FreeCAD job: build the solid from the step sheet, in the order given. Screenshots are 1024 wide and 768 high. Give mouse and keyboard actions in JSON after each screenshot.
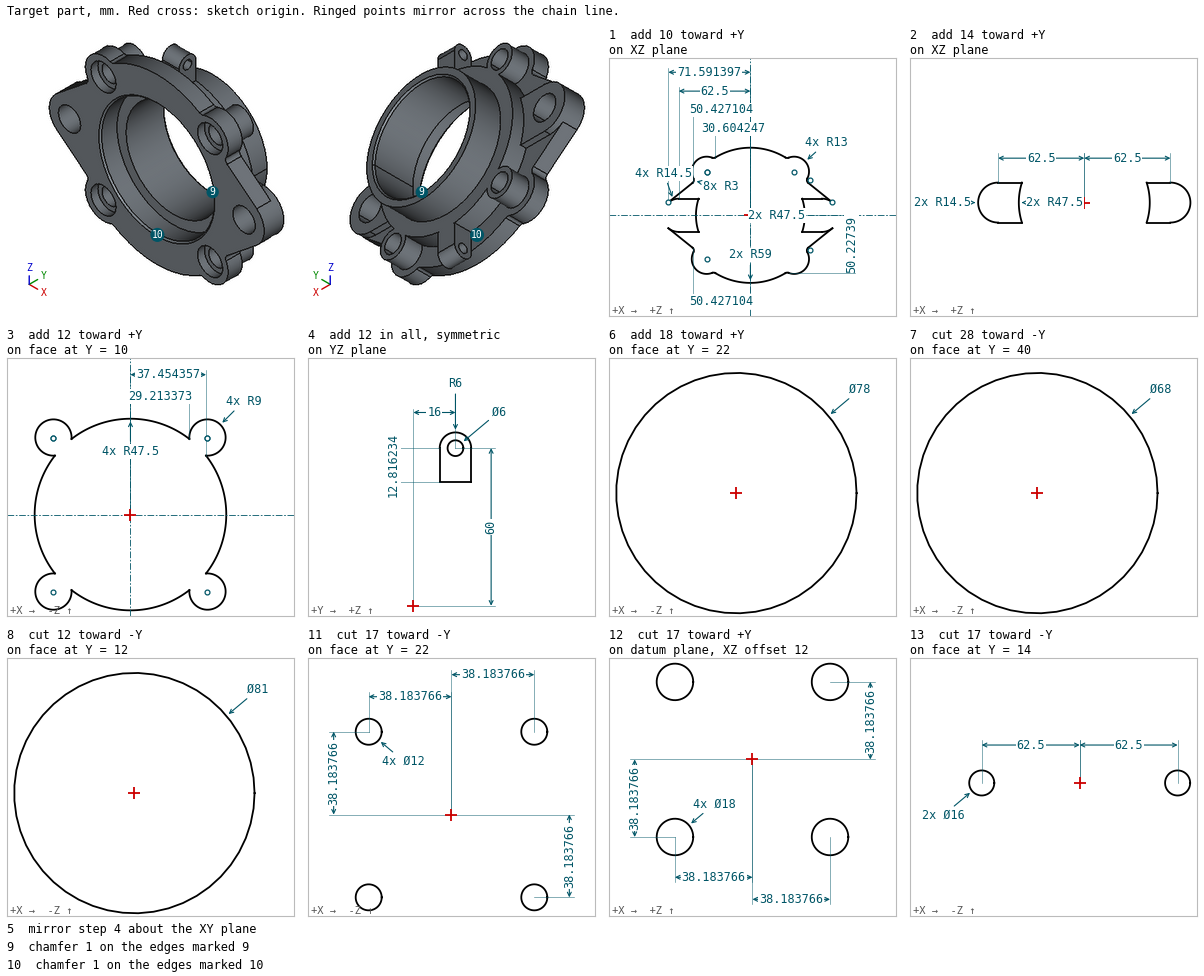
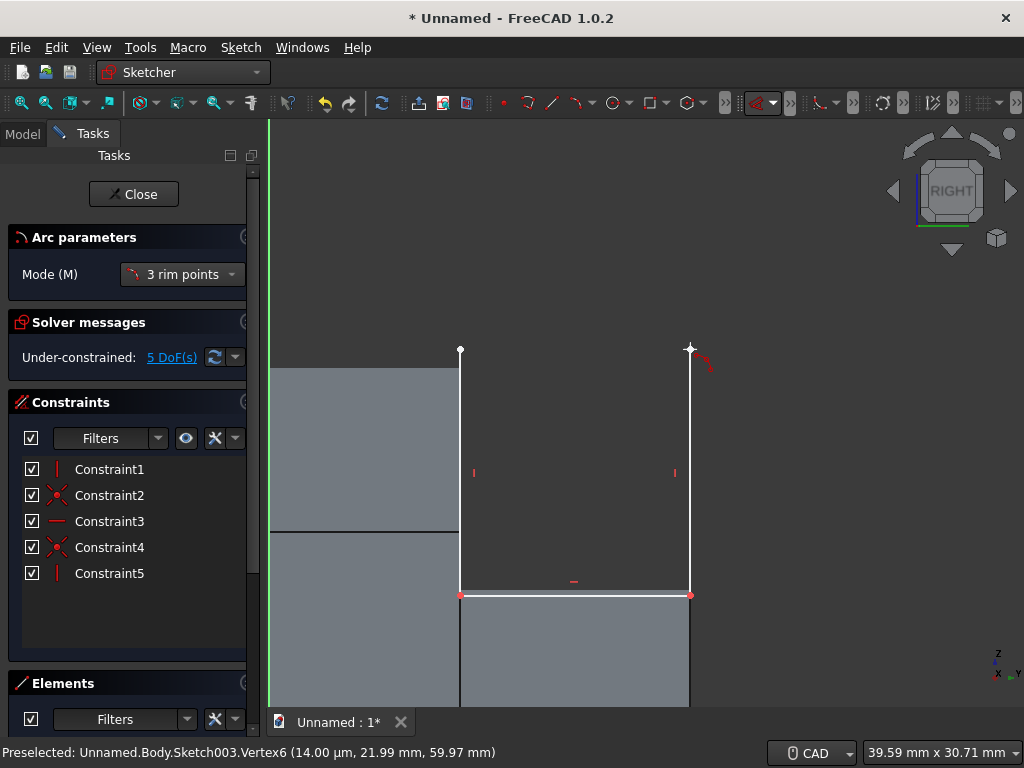
{"action": "left_click", "coordinate": [690, 350]}
{"action": "left_click", "coordinate": [460, 350]}
{"action": "left_click", "coordinate": [575, 234]}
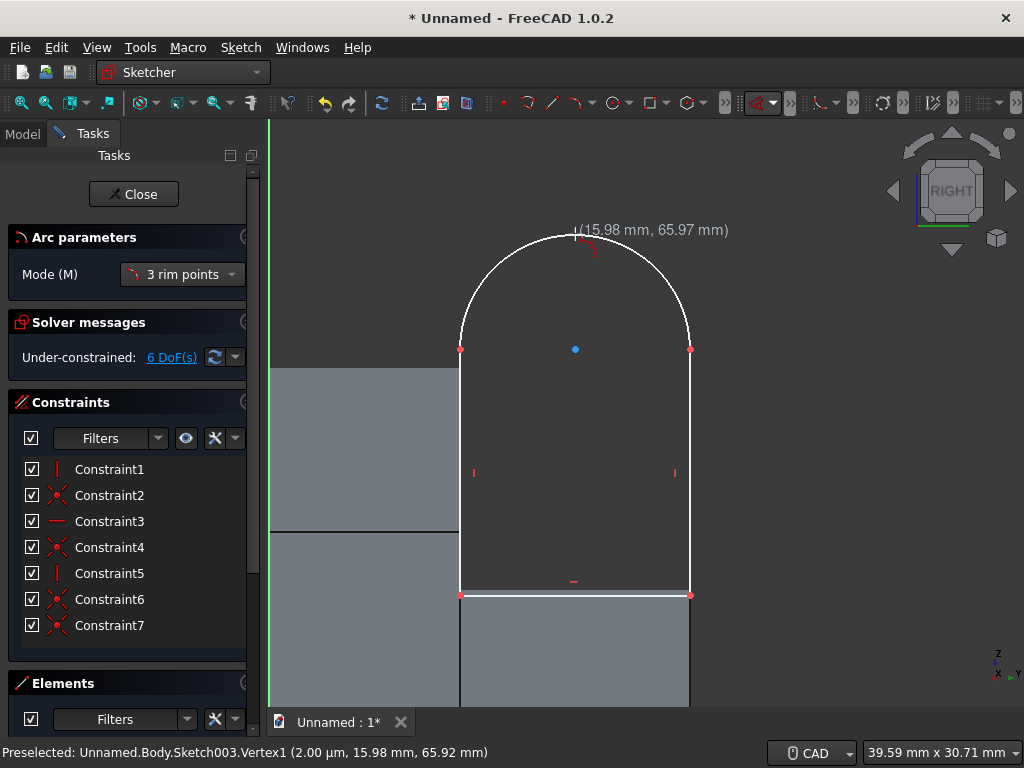
{"action": "key", "text": "g c"}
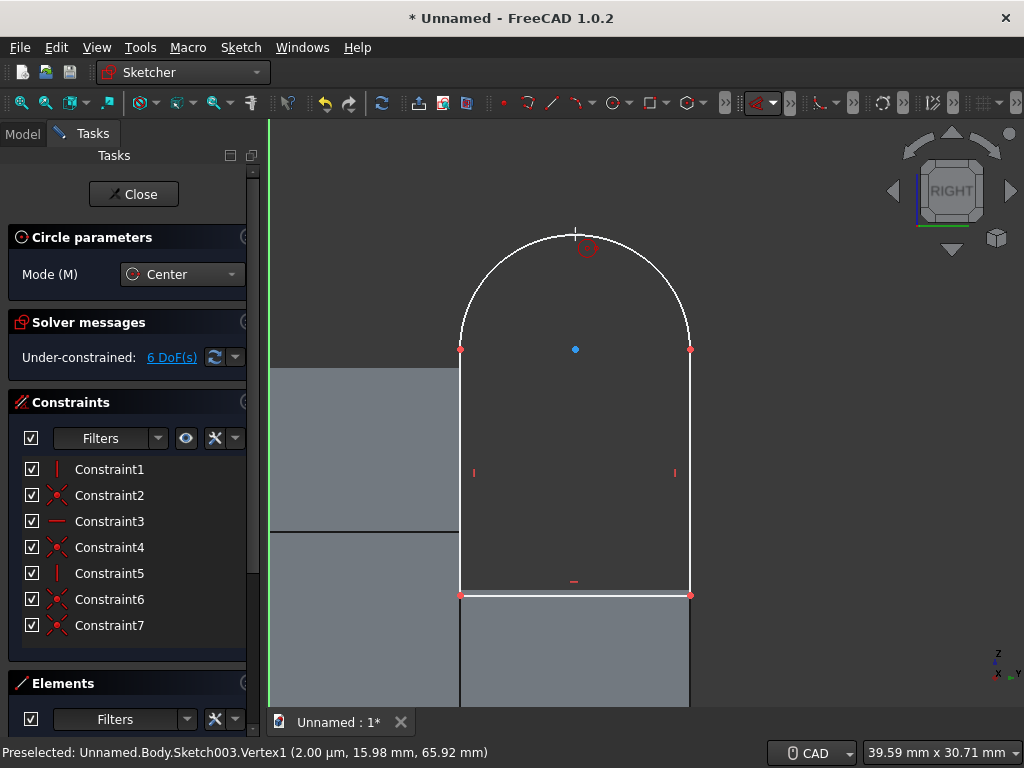
{"action": "left_click", "coordinate": [575, 349]}
{"action": "left_click", "coordinate": [616, 309]}
{"action": "key", "text": "Escape"}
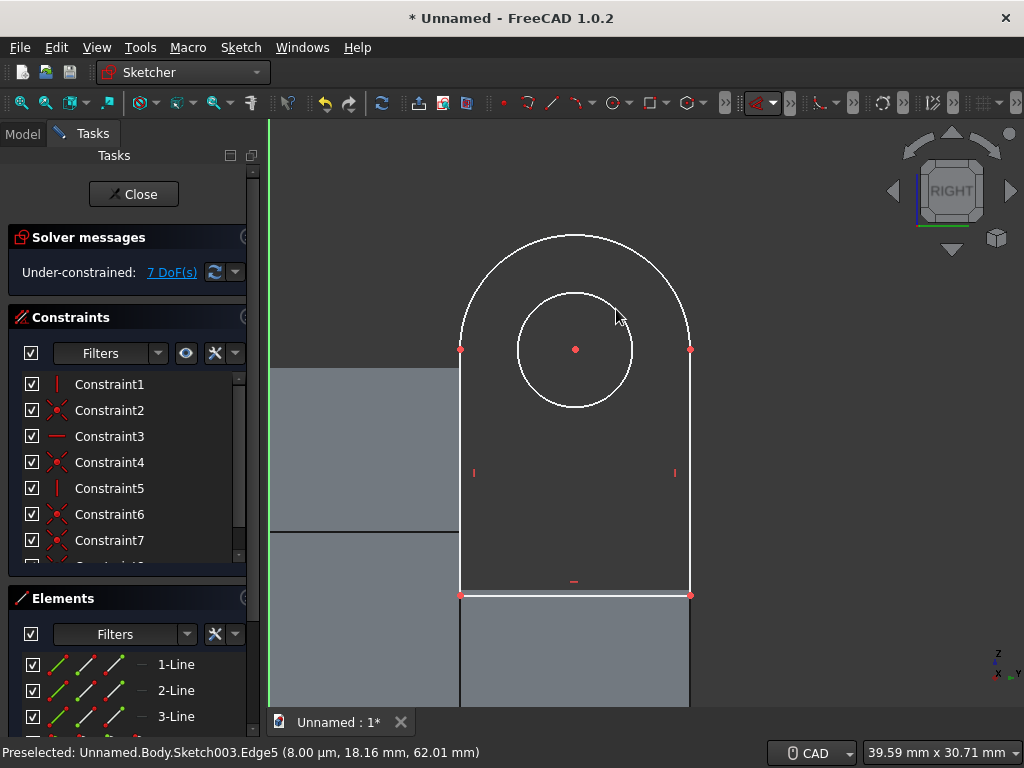
{"action": "left_click", "coordinate": [460, 424]}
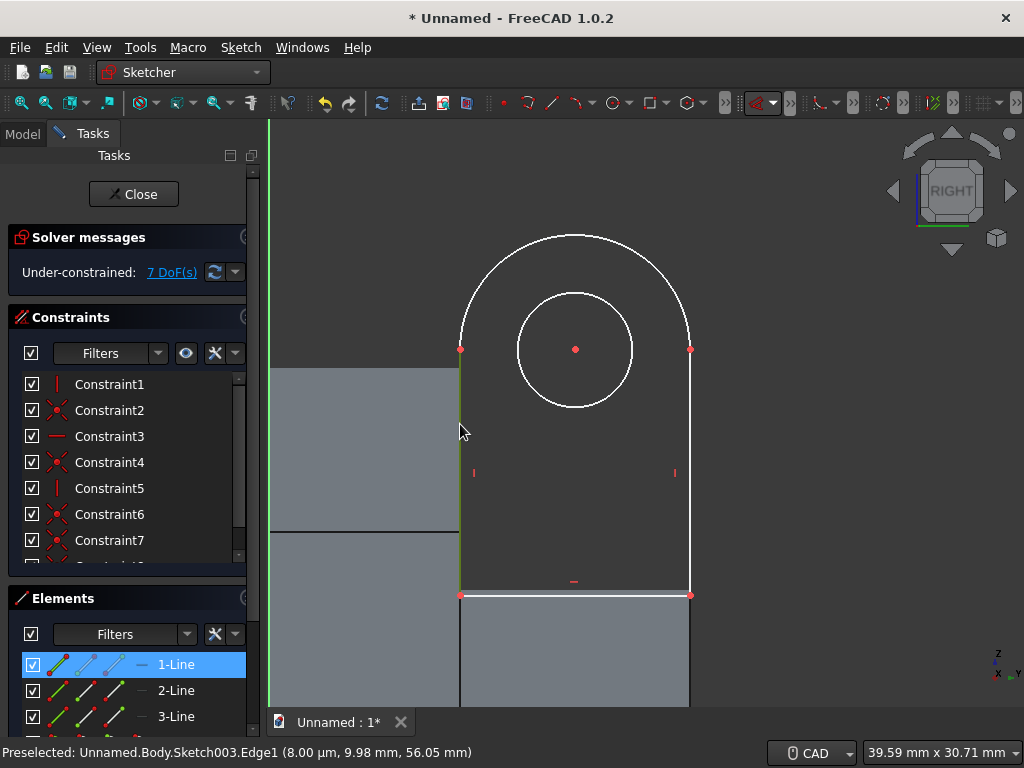
{"action": "left_click", "coordinate": [643, 257]}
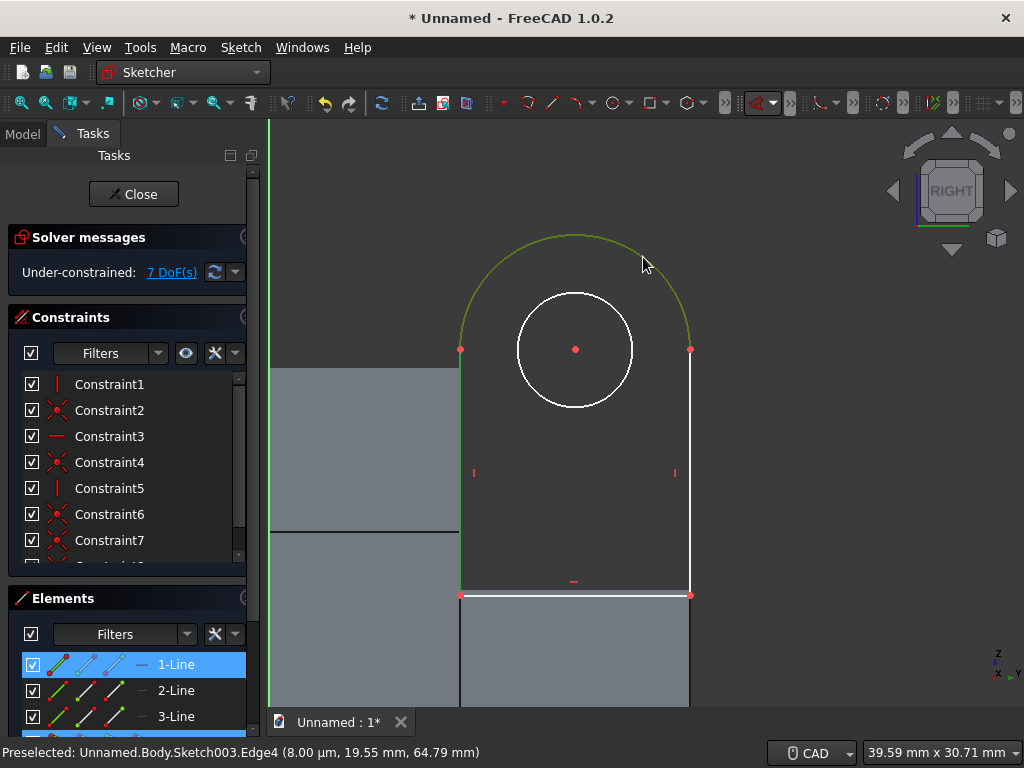
{"action": "key", "text": "t"}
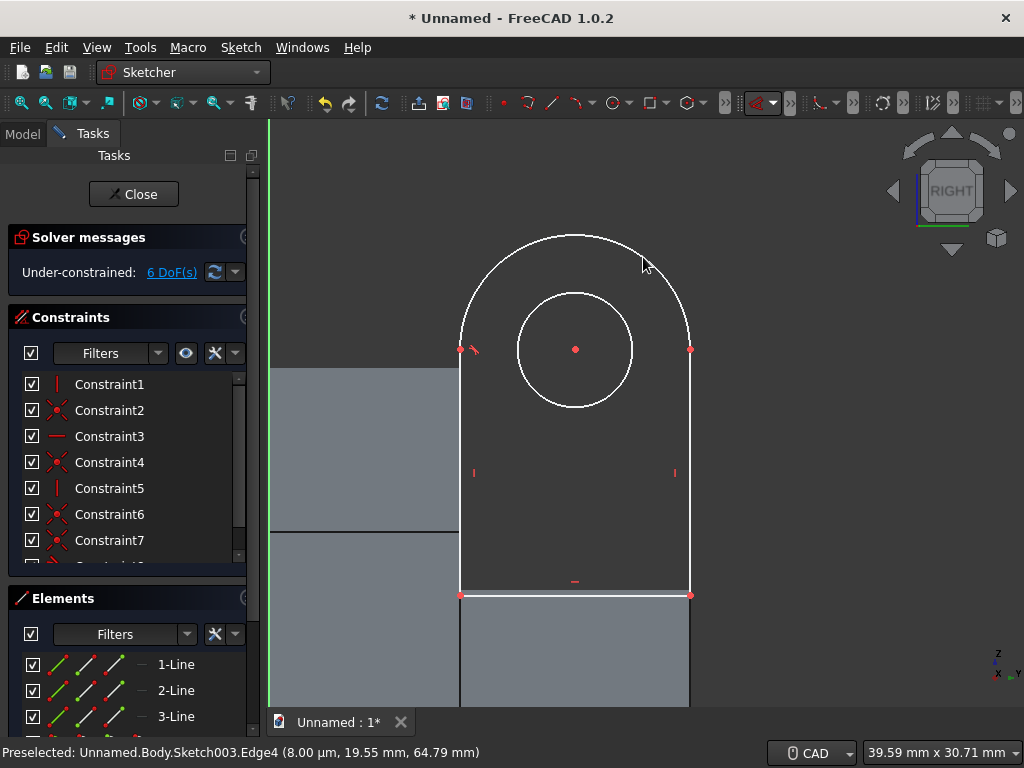
{"action": "left_click", "coordinate": [690, 522]}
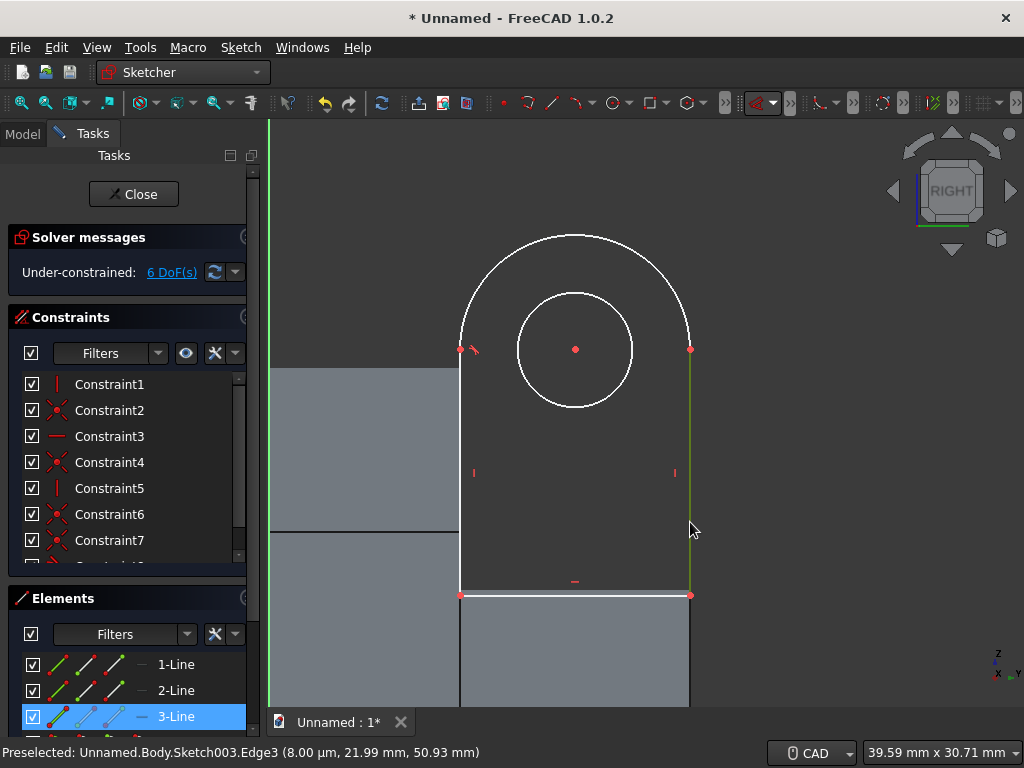
{"action": "left_click", "coordinate": [643, 257]}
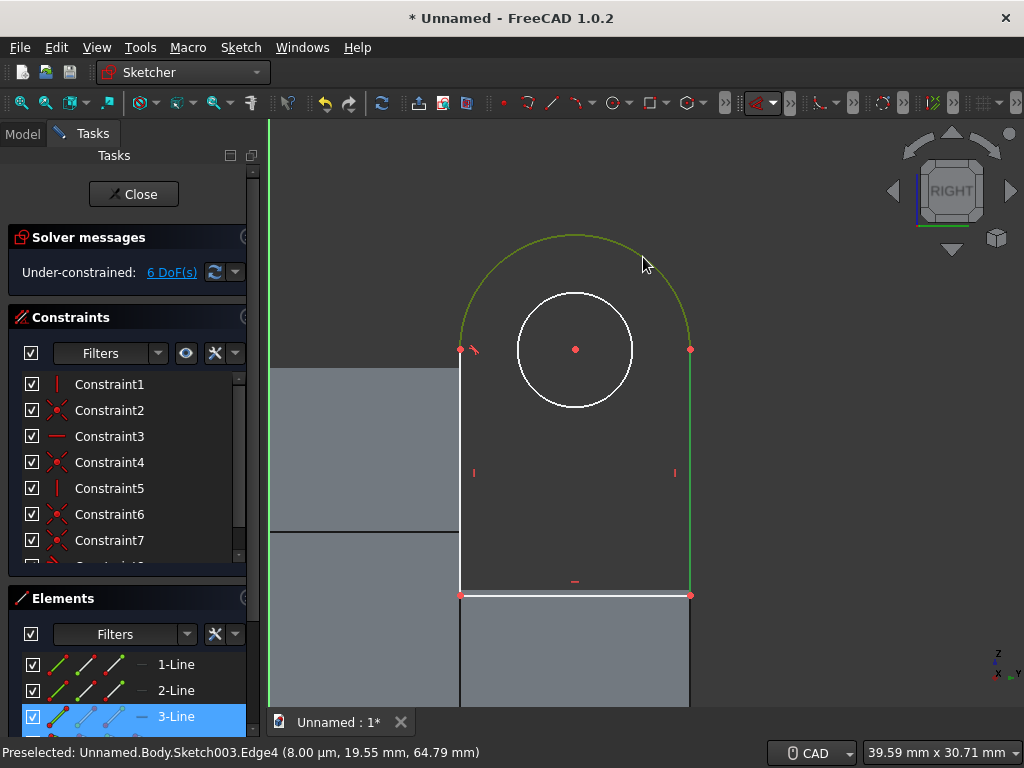
{"action": "key", "text": "t"}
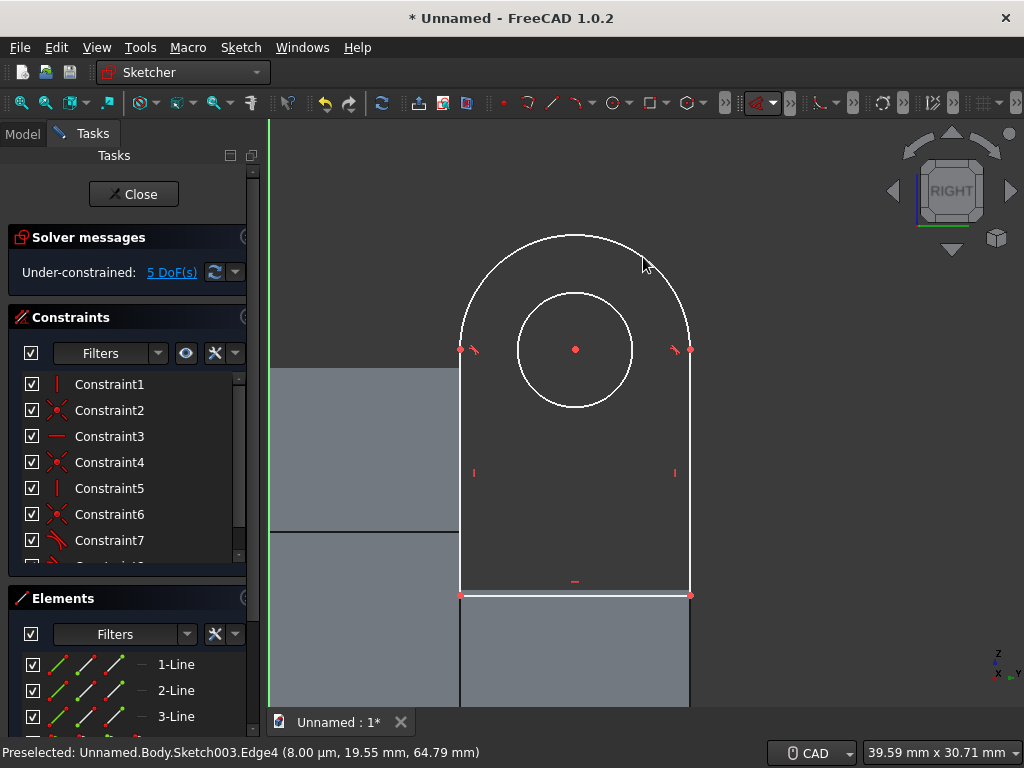
{"action": "key", "text": "d"}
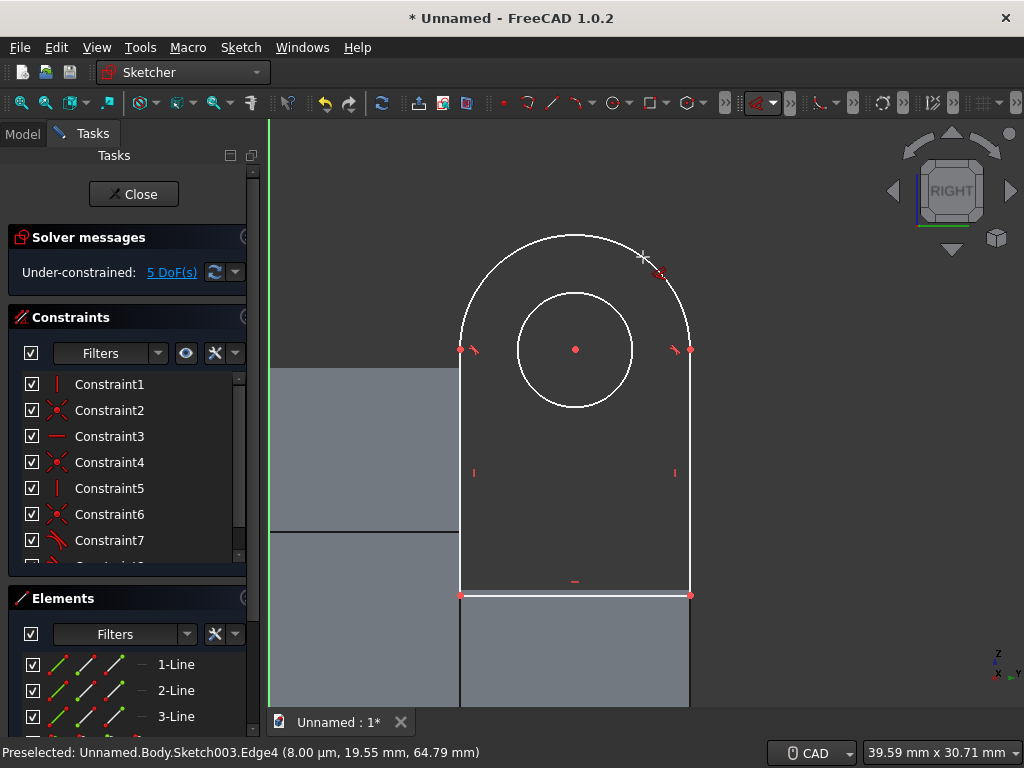
{"action": "left_click", "coordinate": [643, 257]}
{"action": "left_click", "coordinate": [662, 231]}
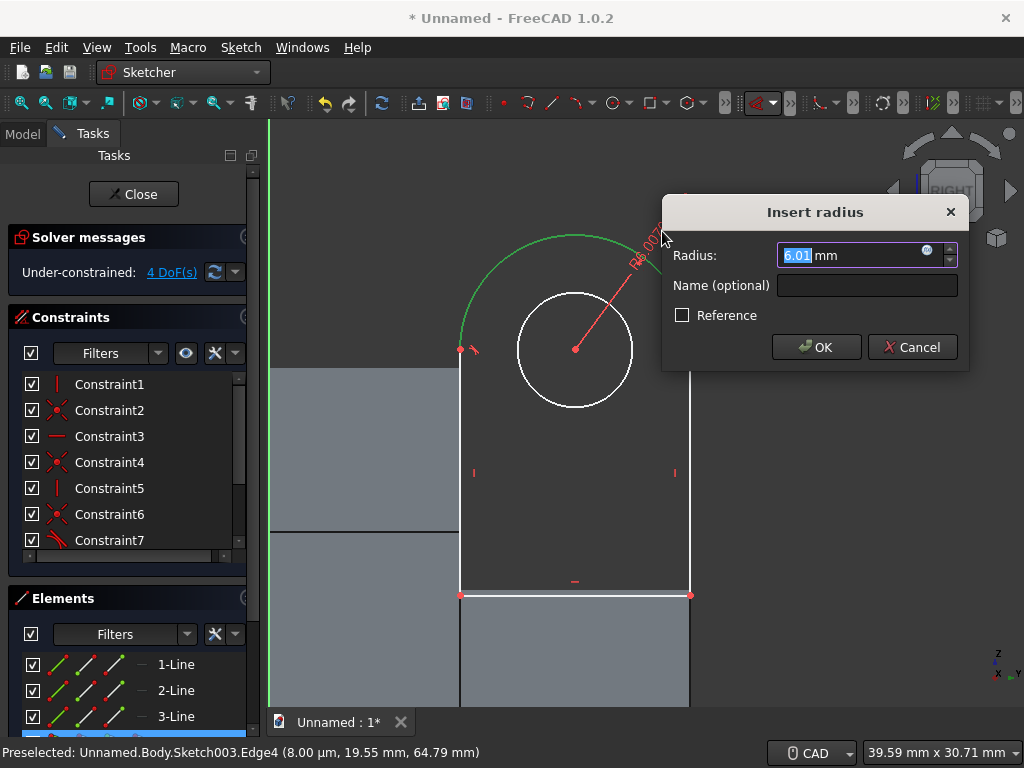
{"action": "type", "text": "6"}
{"action": "key", "text": "Return"}